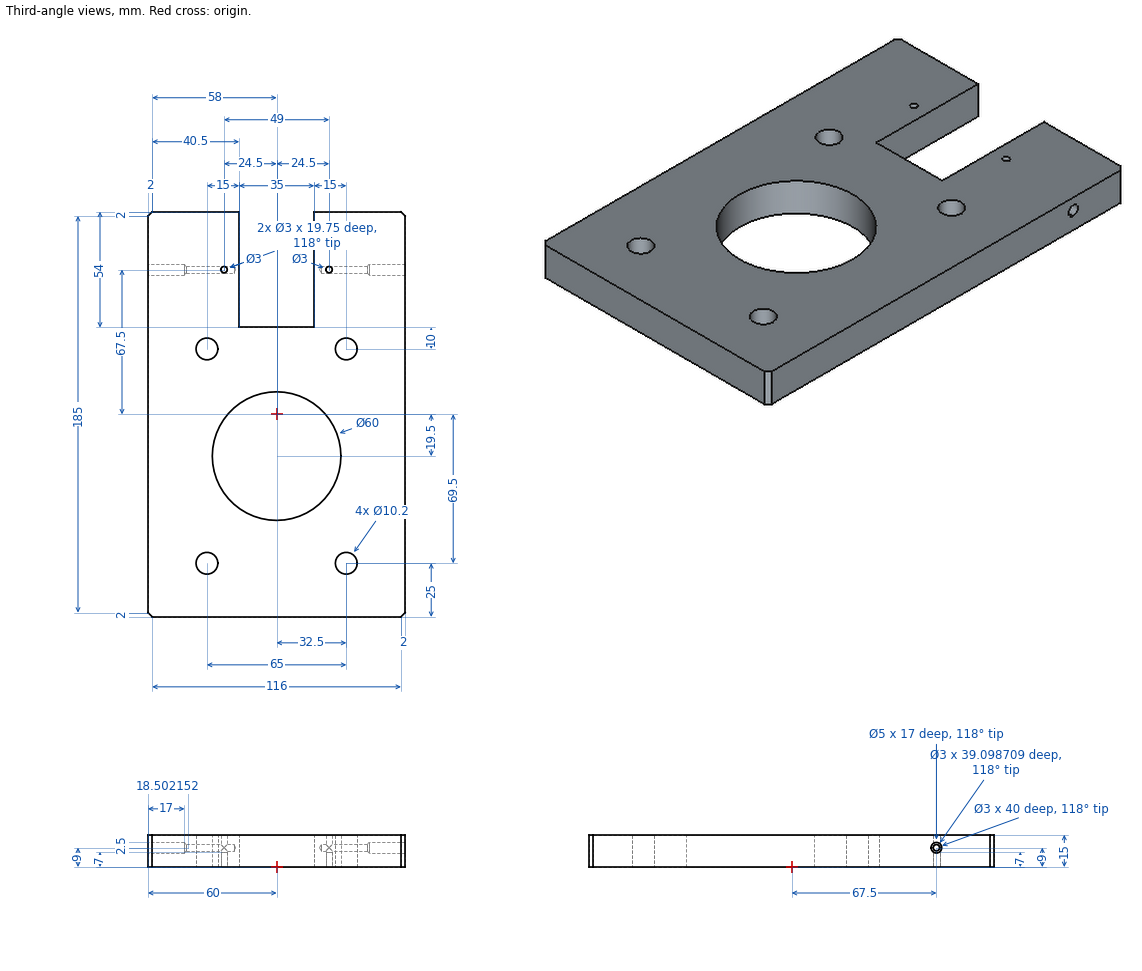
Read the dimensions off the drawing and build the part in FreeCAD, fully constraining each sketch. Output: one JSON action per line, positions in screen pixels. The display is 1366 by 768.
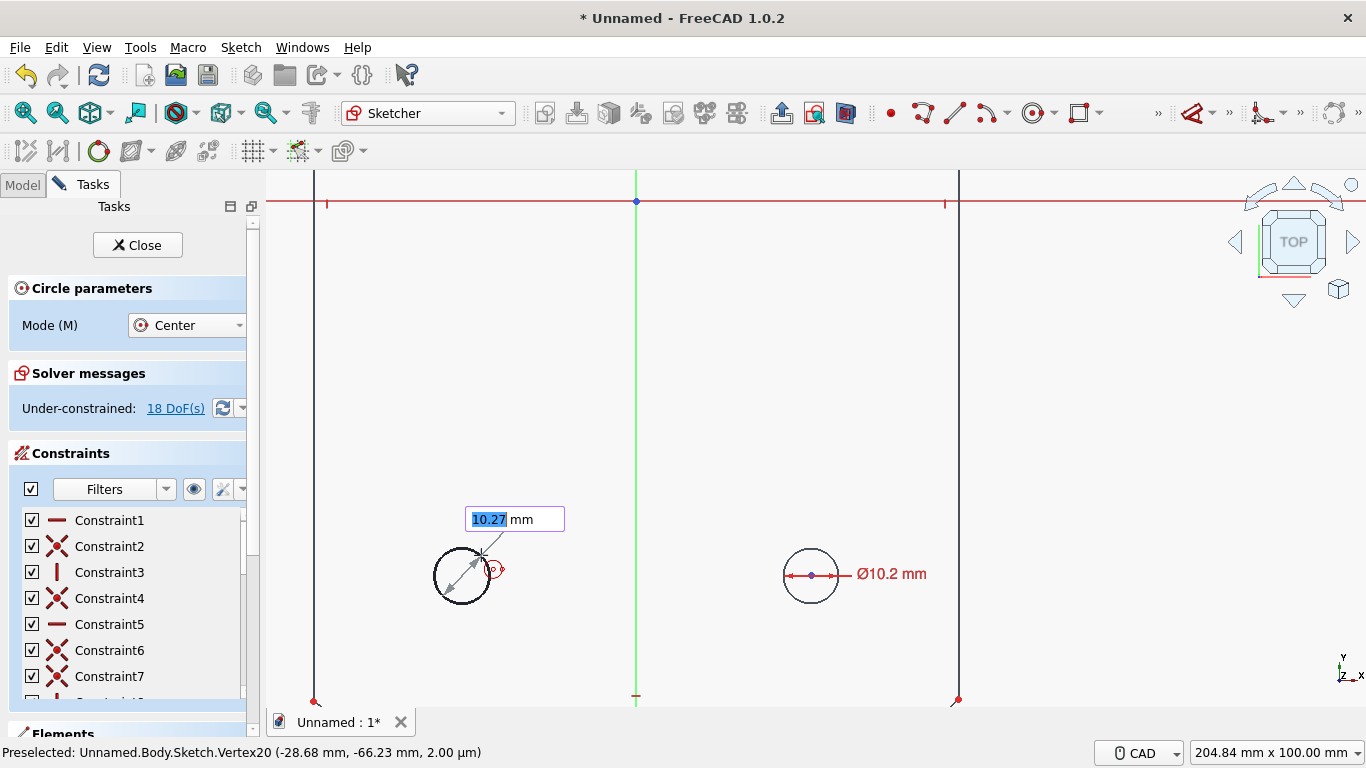
{"action": "type", "text": "10.2"}
{"action": "key", "text": "Return"}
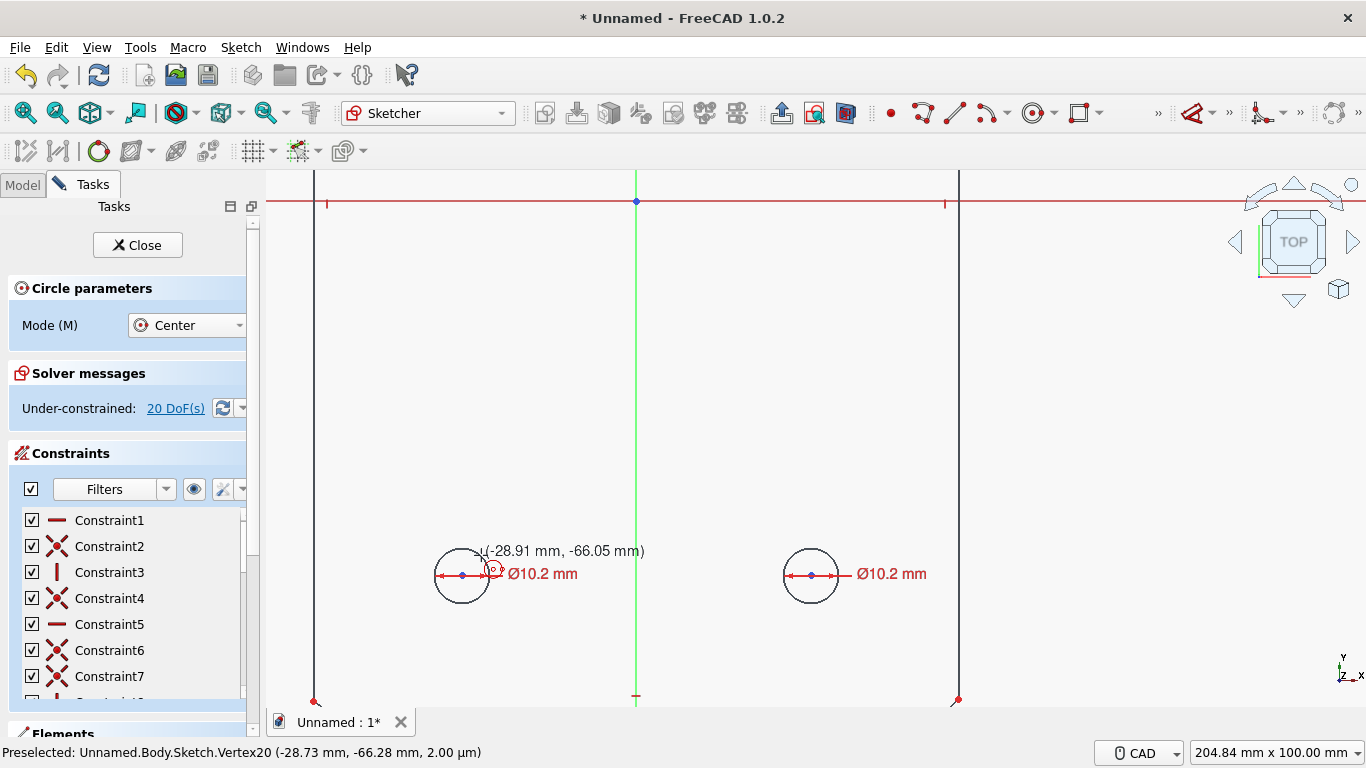
{"action": "scroll", "coordinate": [812, 577], "scroll_direction": "down", "scroll_amount": 5}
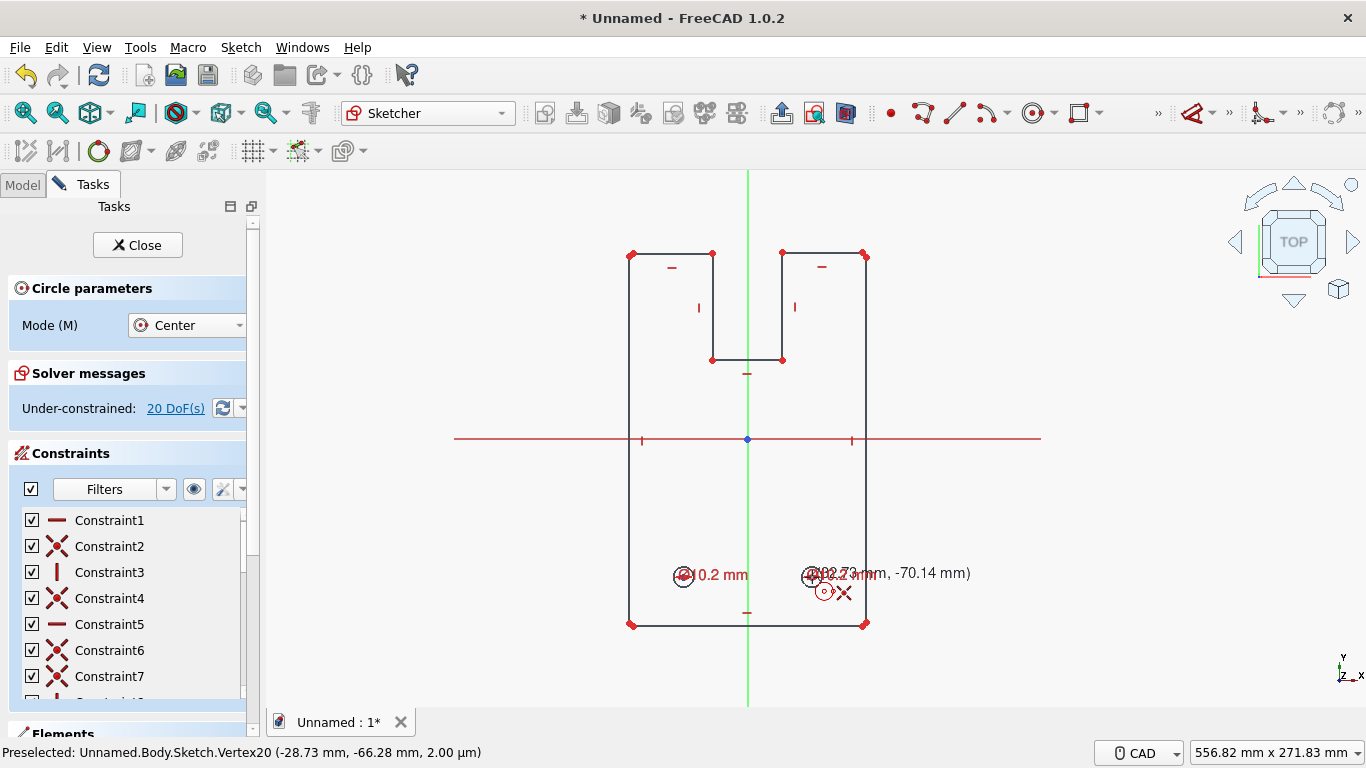
{"action": "scroll", "coordinate": [812, 379], "scroll_direction": "up", "scroll_amount": 5}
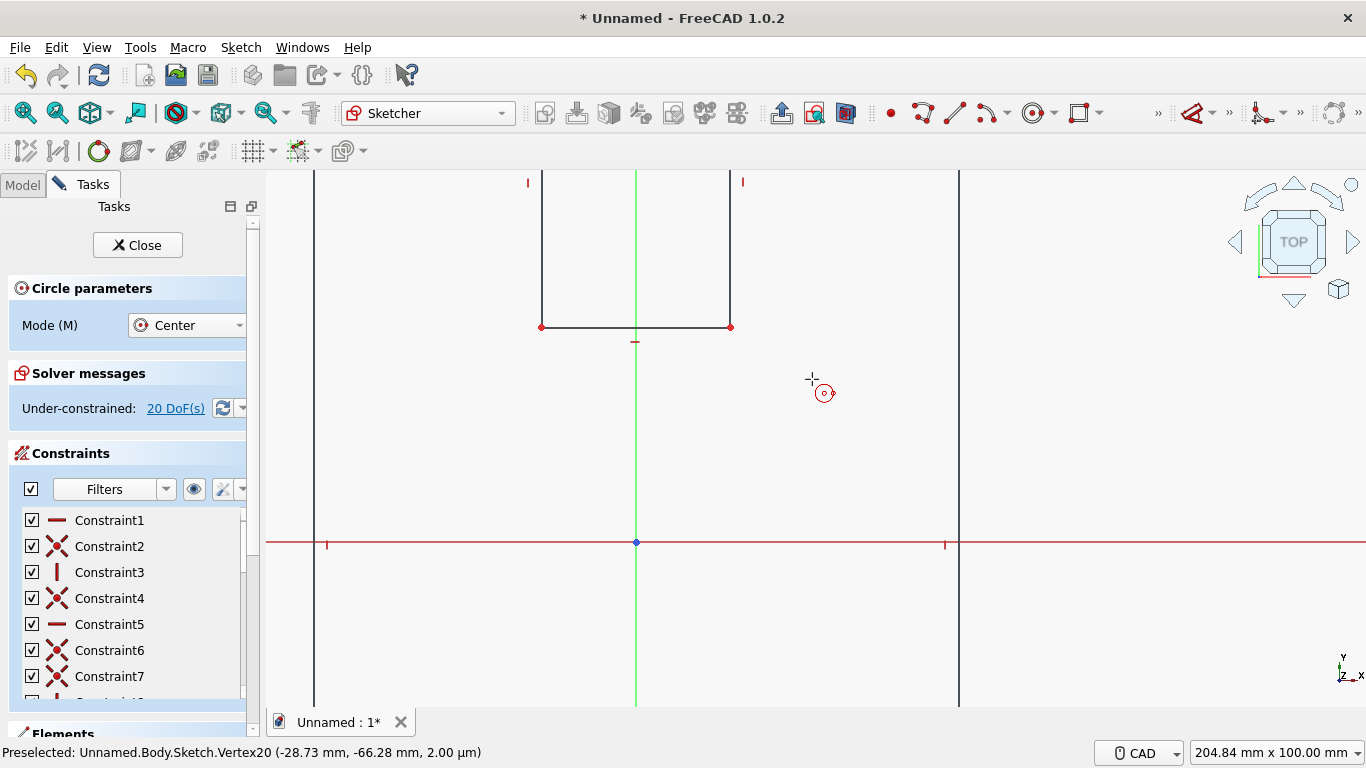
{"action": "left_click", "coordinate": [811, 378]}
{"action": "mouse_move", "coordinate": [830, 359]}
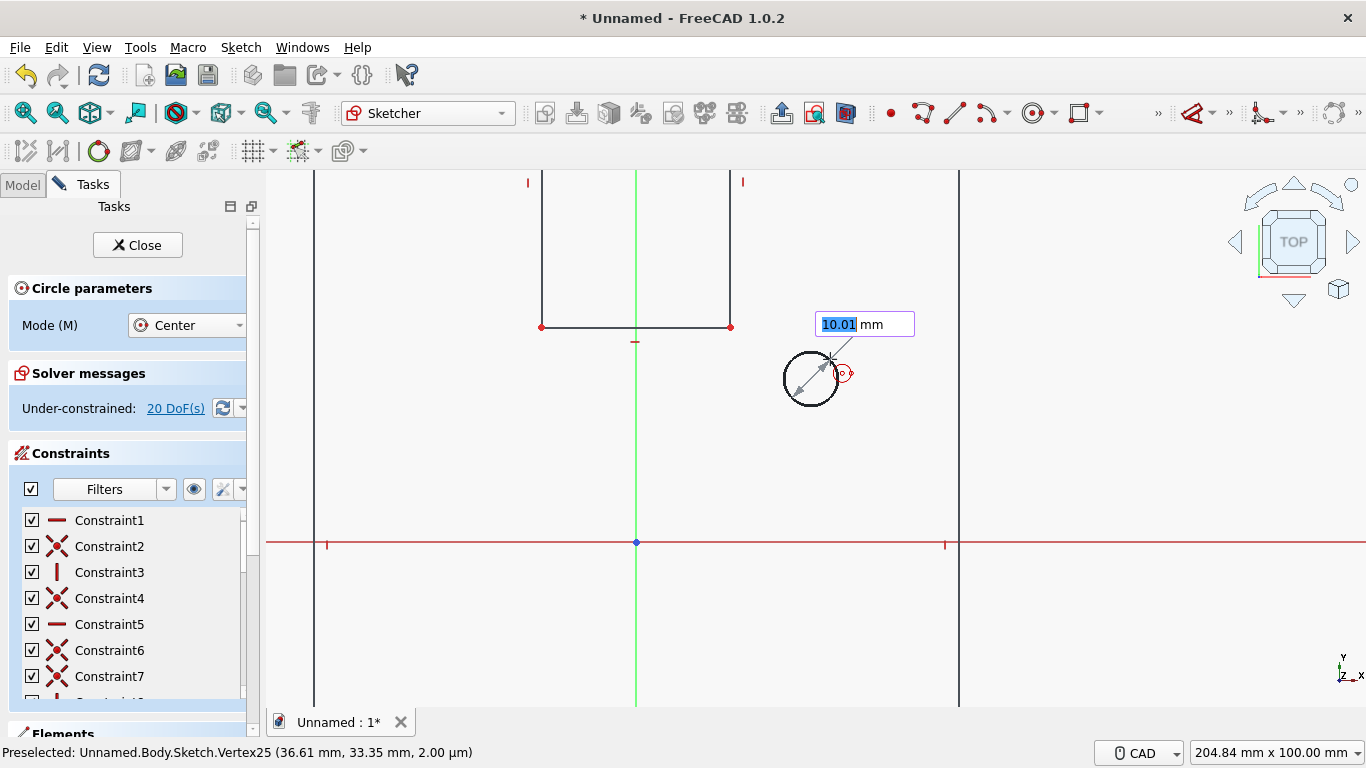
{"action": "type", "text": "10.2"}
{"action": "key", "text": "Return"}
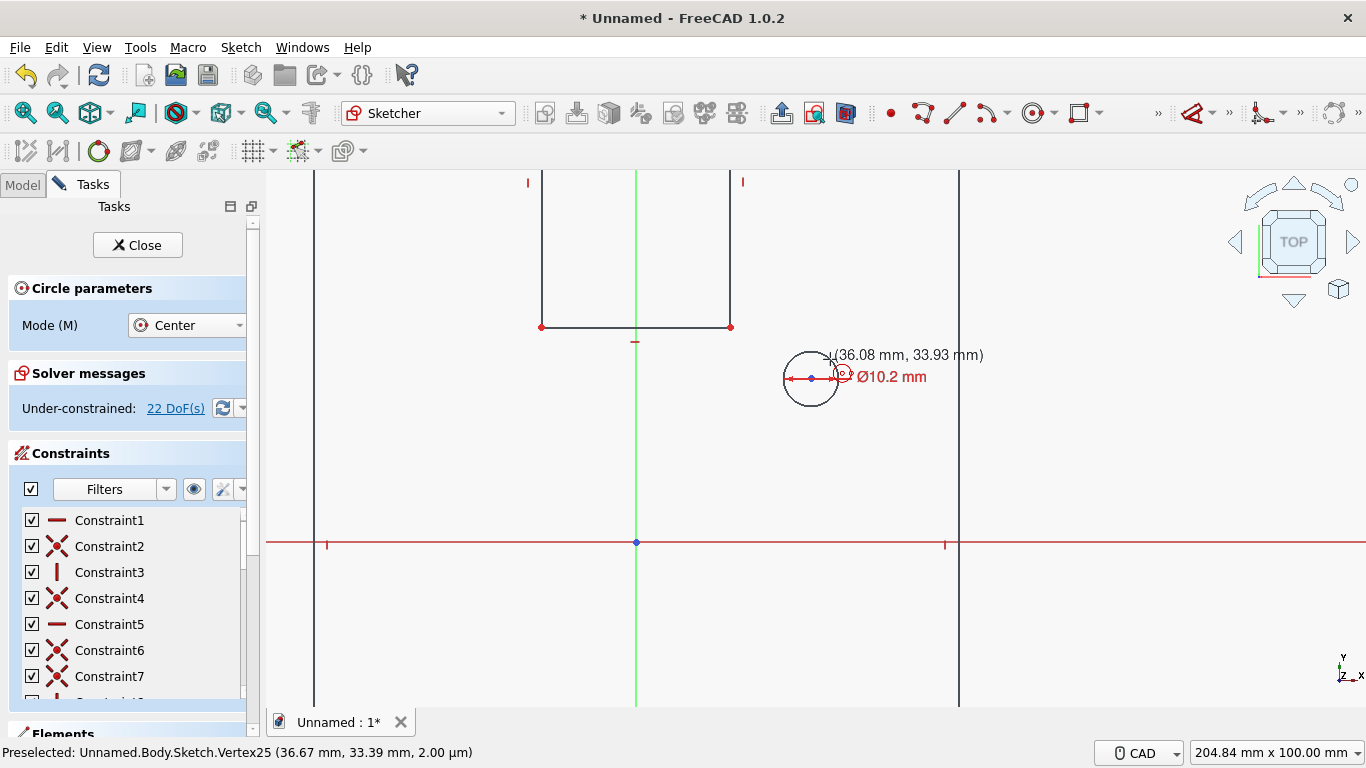
{"action": "left_click", "coordinate": [462, 378]}
{"action": "mouse_move", "coordinate": [481, 359]}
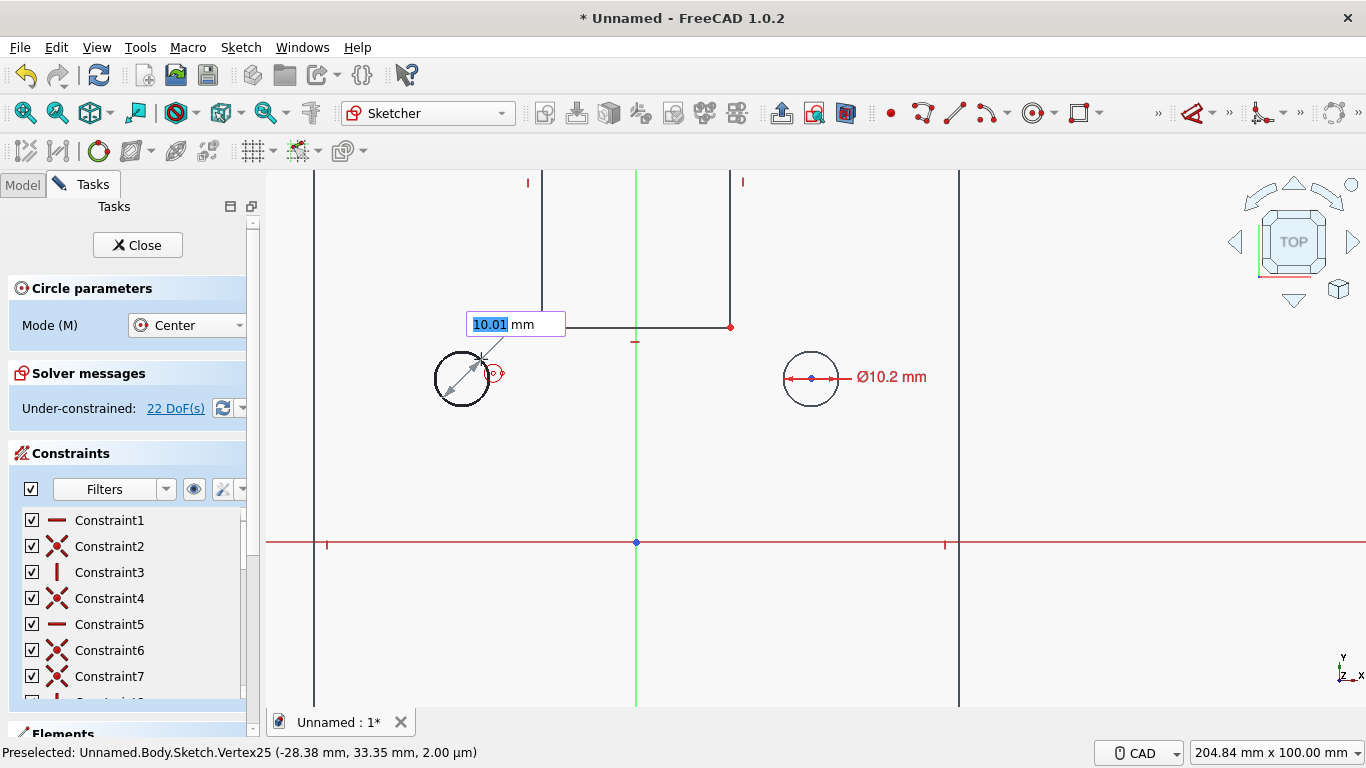
{"action": "type", "text": "10.2"}
{"action": "key", "text": "Return"}
{"action": "key", "text": "Escape"}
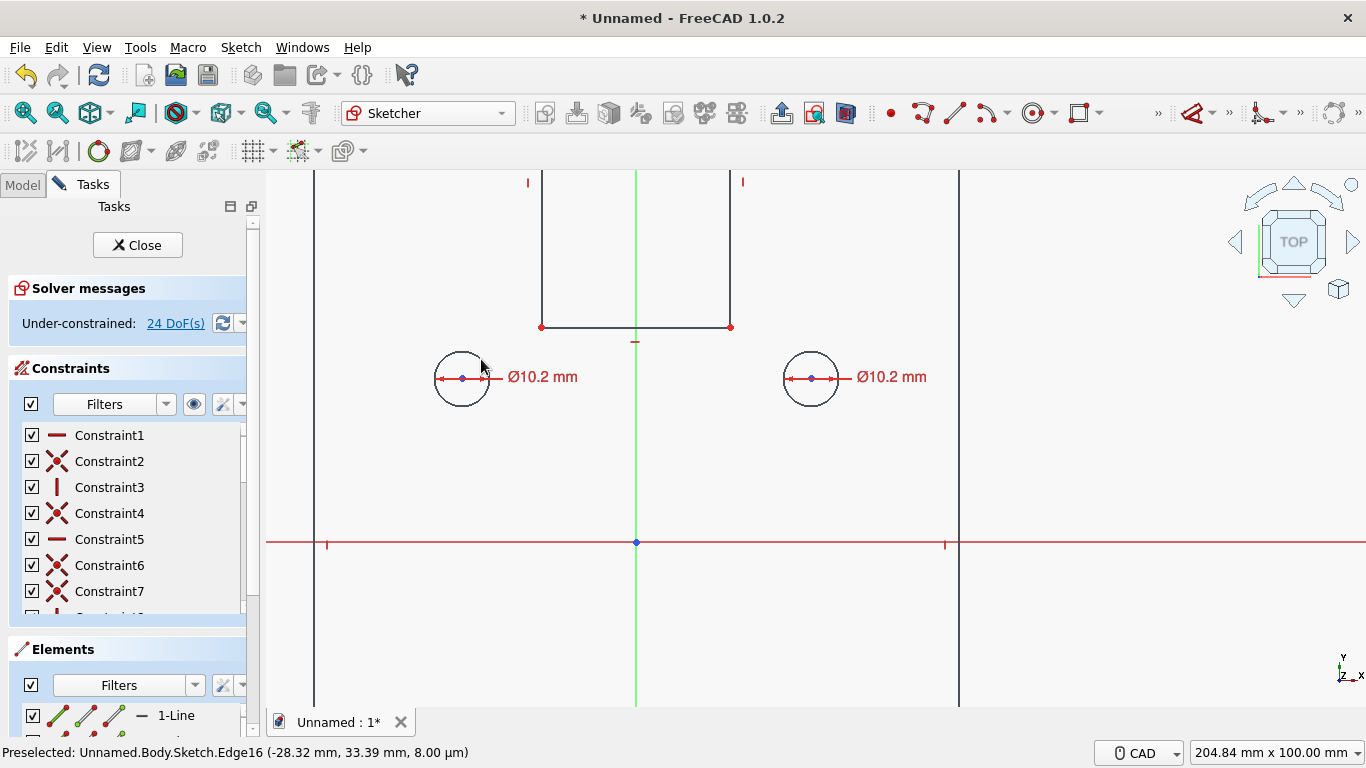
{"action": "left_click", "coordinate": [674, 328]}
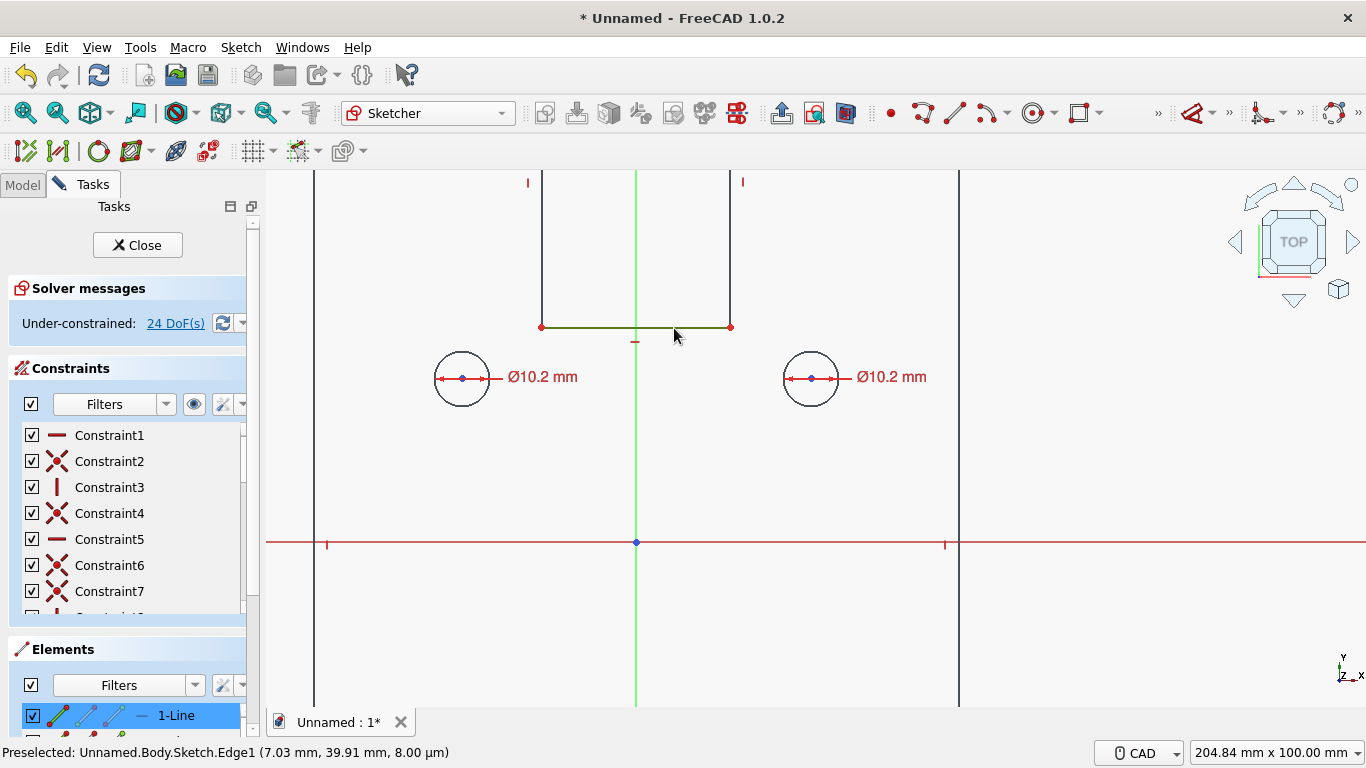
{"action": "key", "text": "l"}